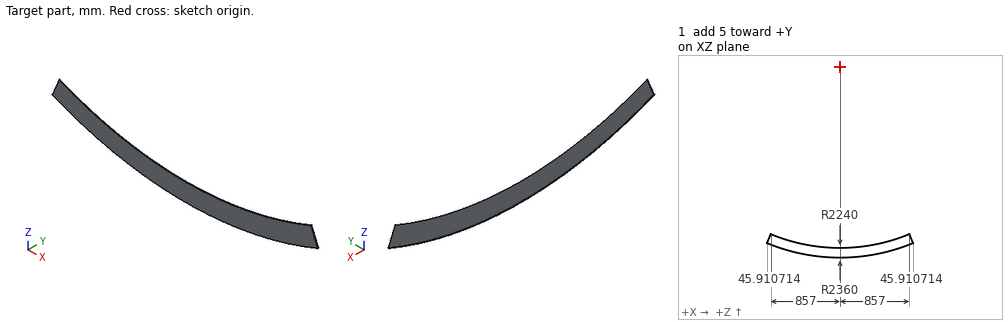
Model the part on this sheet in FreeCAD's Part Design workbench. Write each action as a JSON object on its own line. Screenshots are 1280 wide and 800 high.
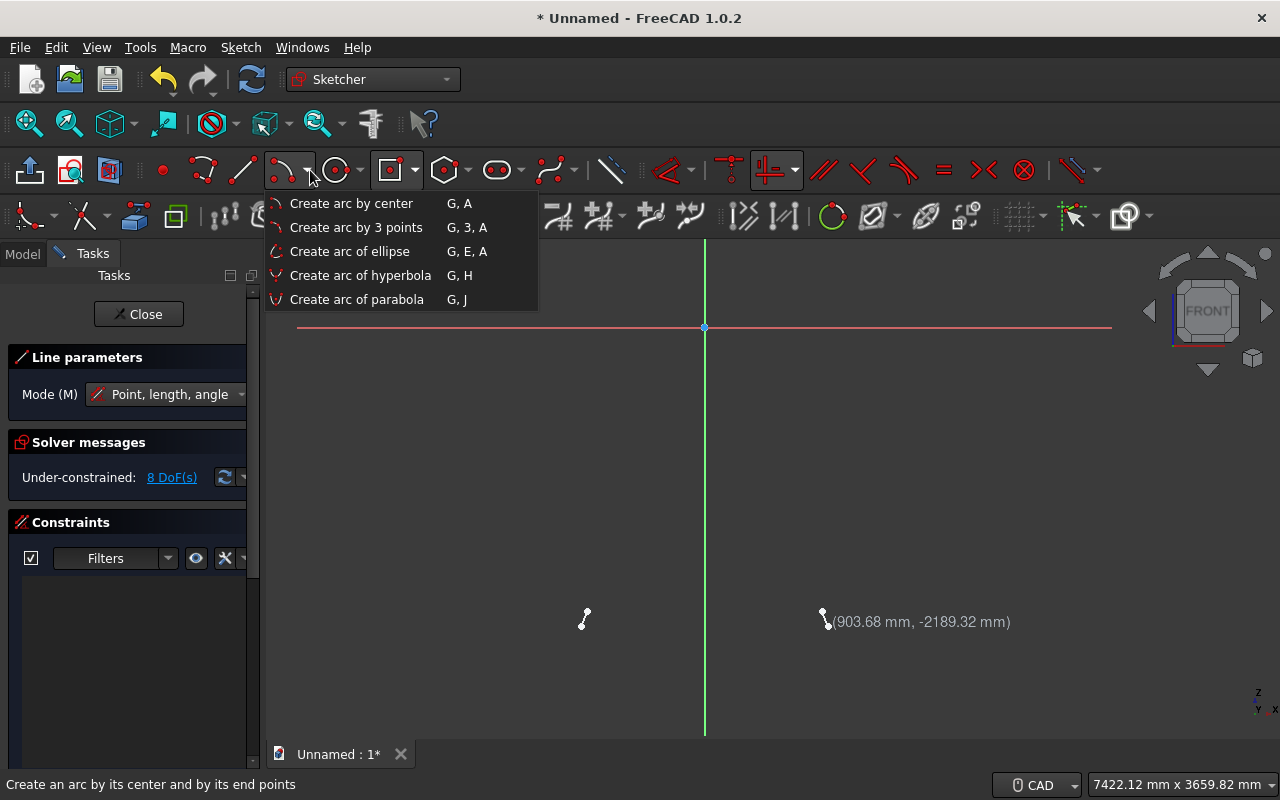
{"action": "left_click", "coordinate": [402, 227]}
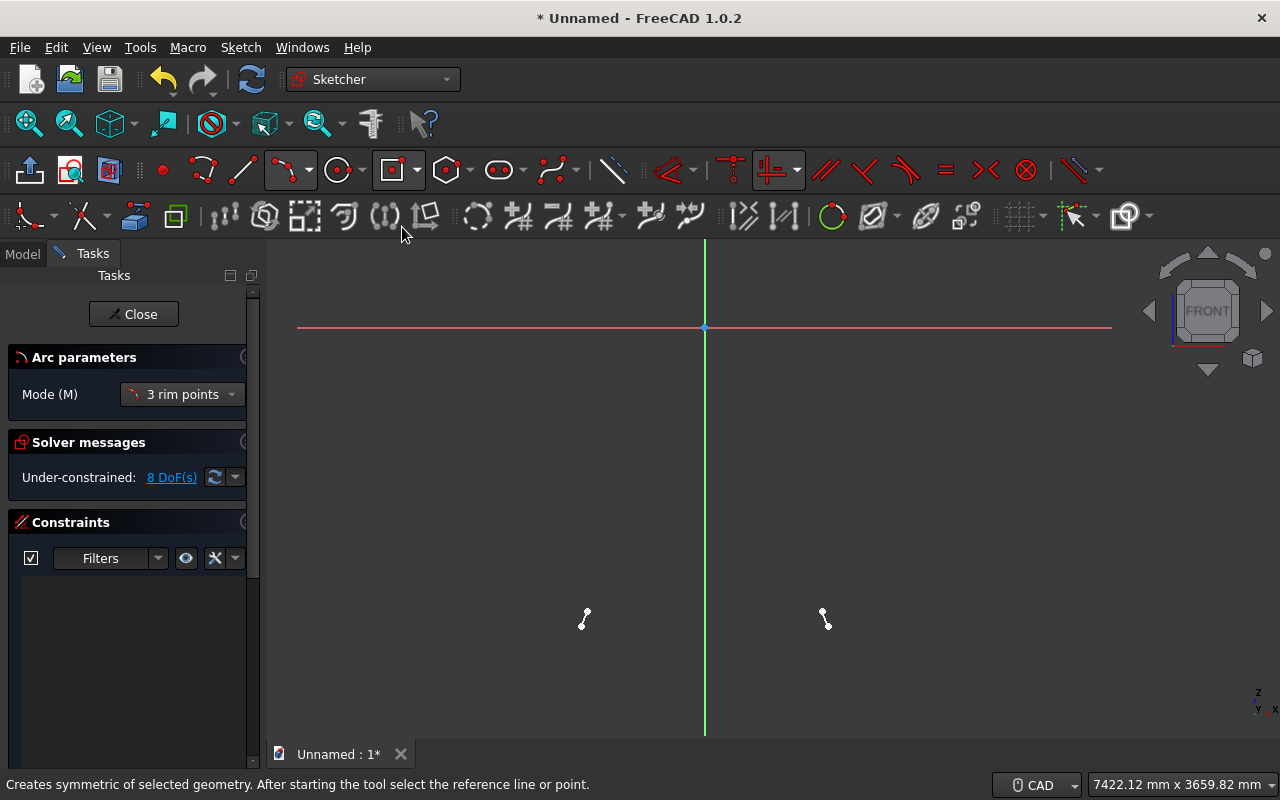
{"action": "scroll", "coordinate": [587, 611], "scroll_direction": "up", "scroll_amount": 4}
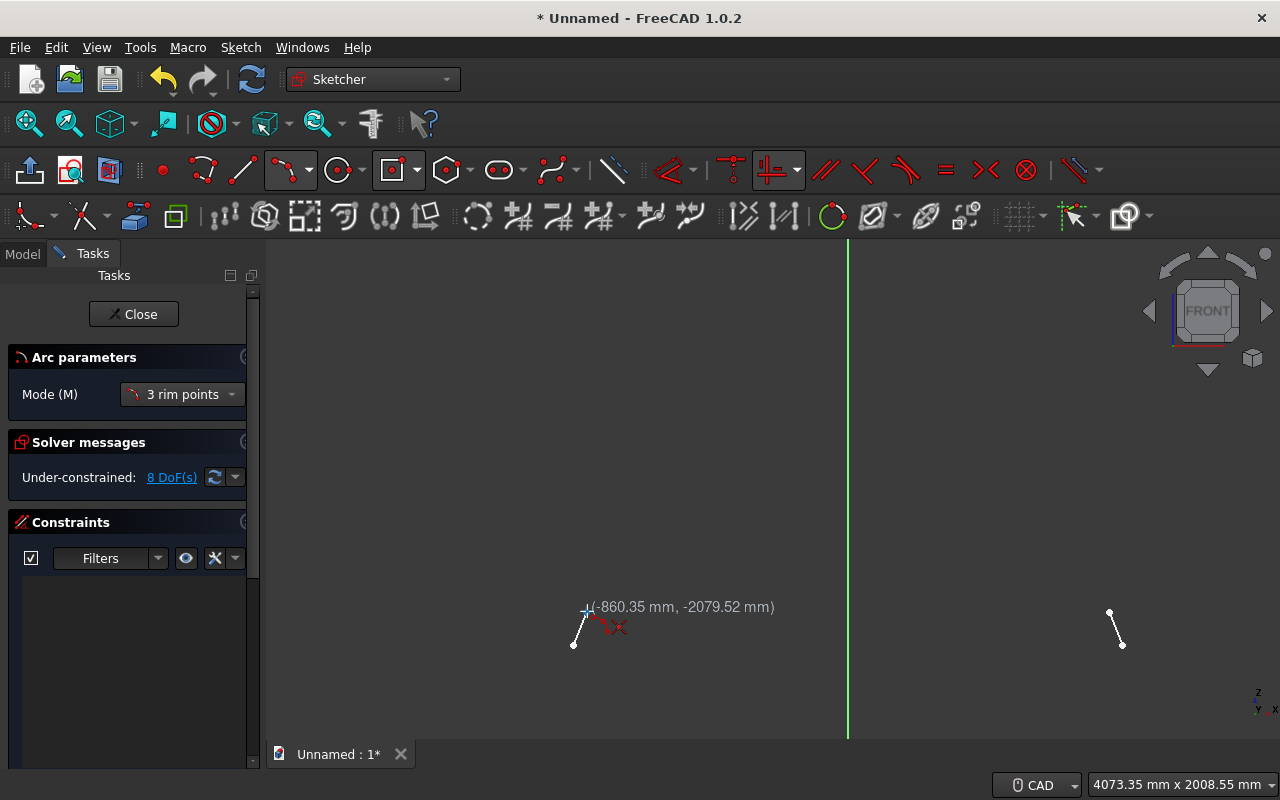
{"action": "left_click", "coordinate": [587, 612]}
{"action": "left_click", "coordinate": [1110, 612]}
{"action": "left_click", "coordinate": [795, 659]}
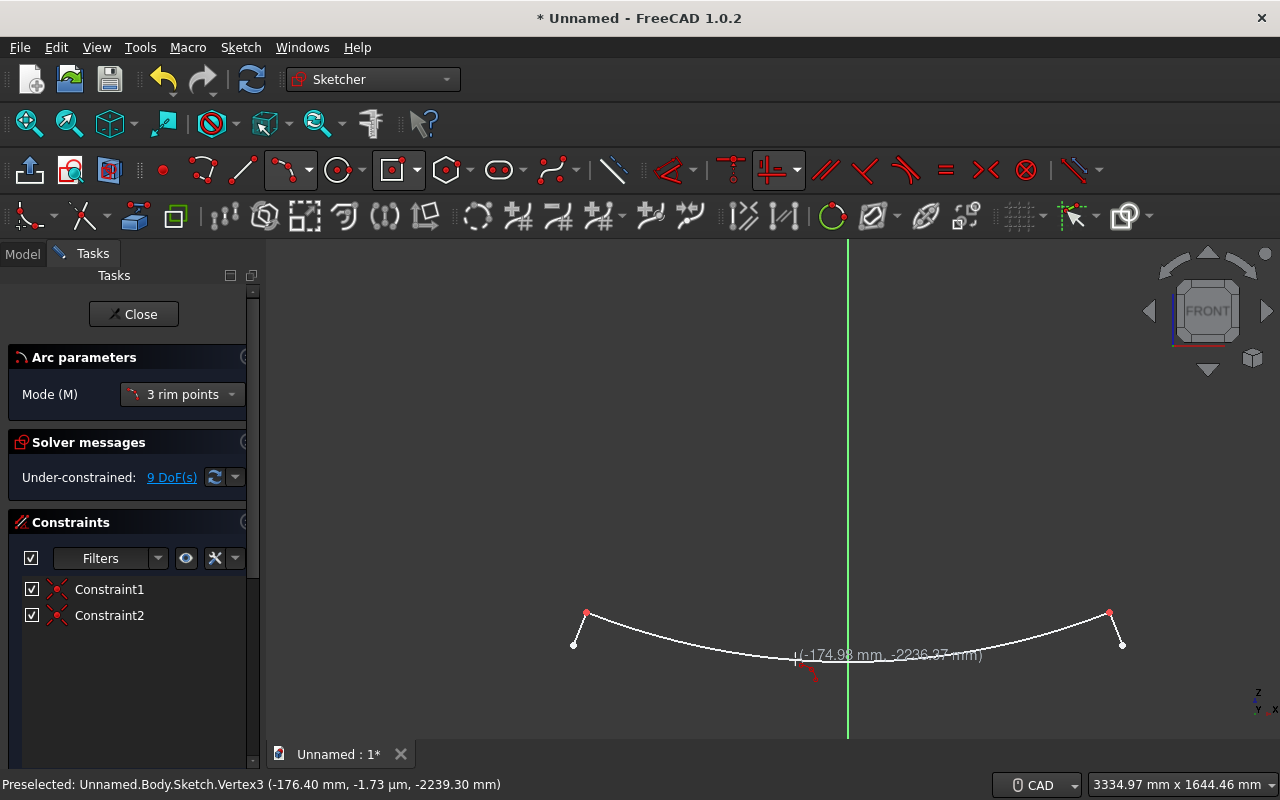
{"action": "scroll", "coordinate": [587, 612], "scroll_direction": "down", "scroll_amount": 4}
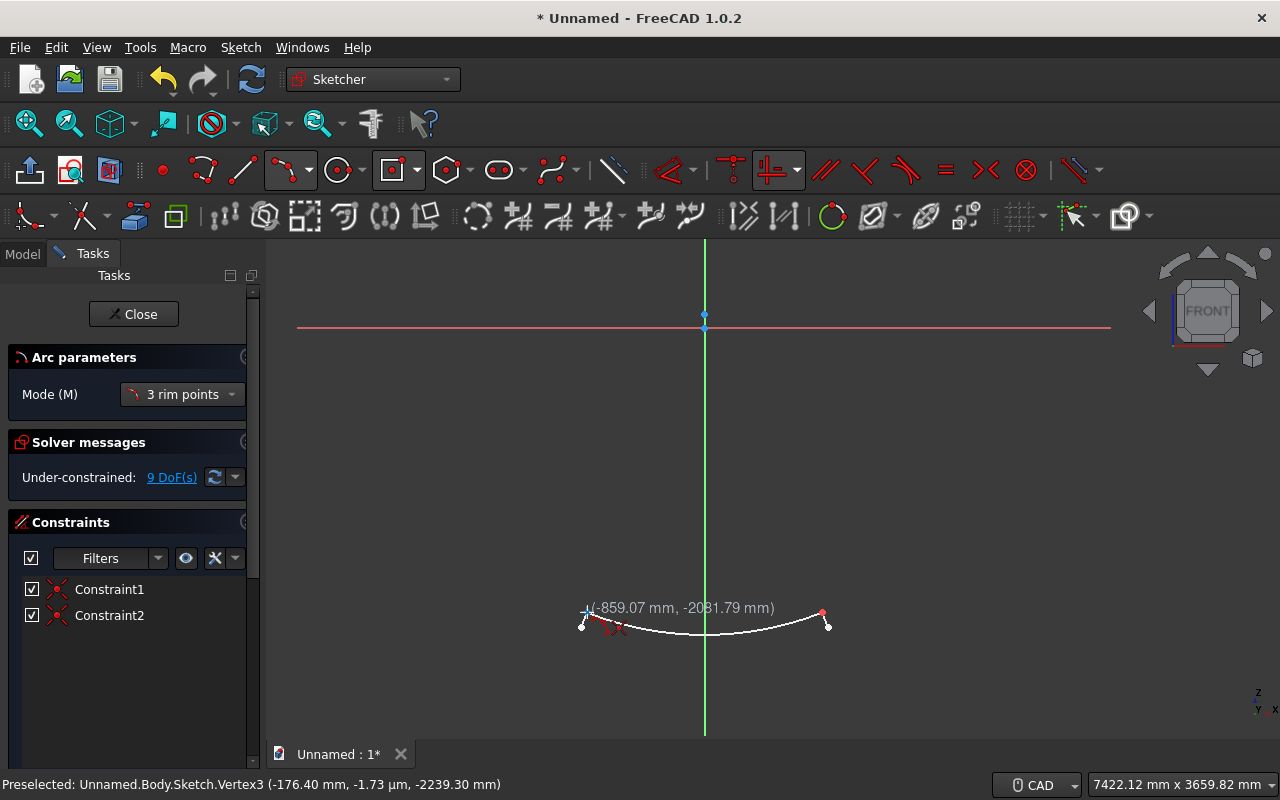
{"action": "scroll", "coordinate": [828, 626], "scroll_direction": "up", "scroll_amount": 4}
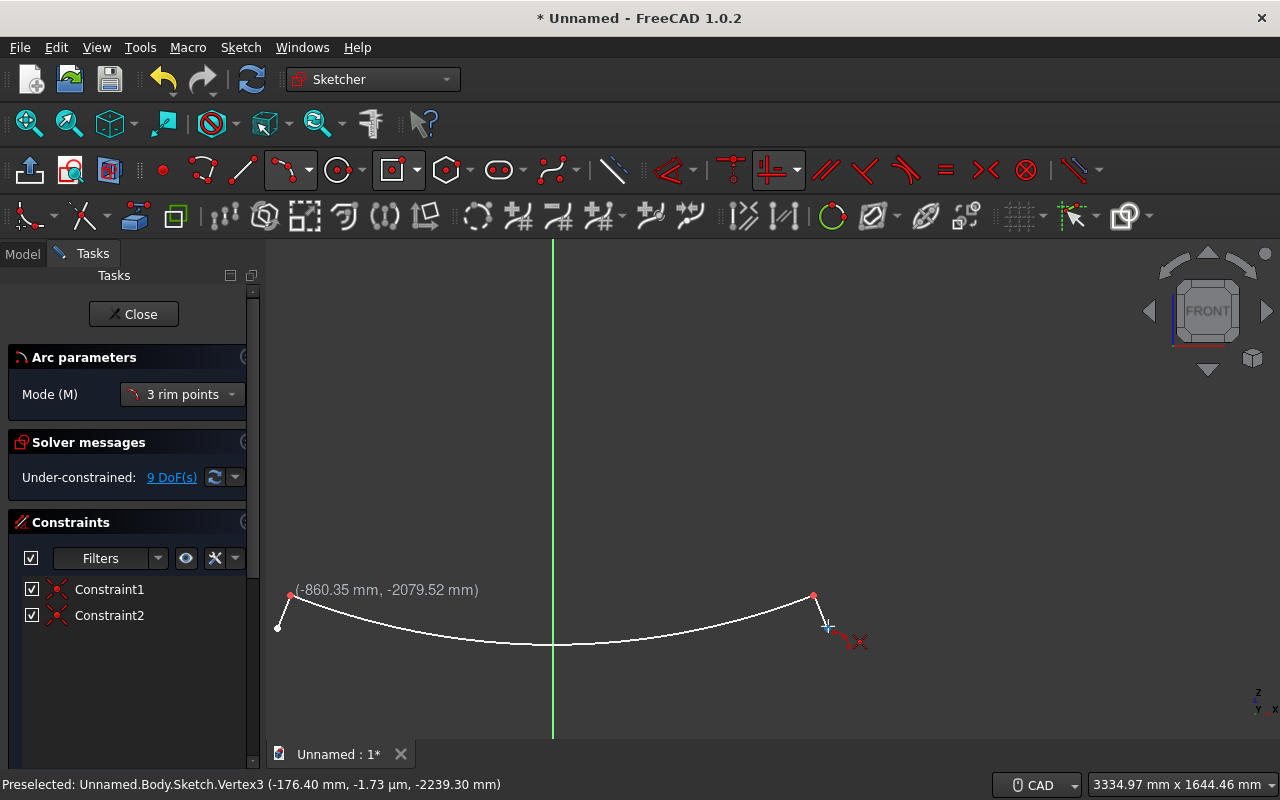
{"action": "left_click", "coordinate": [827, 629]}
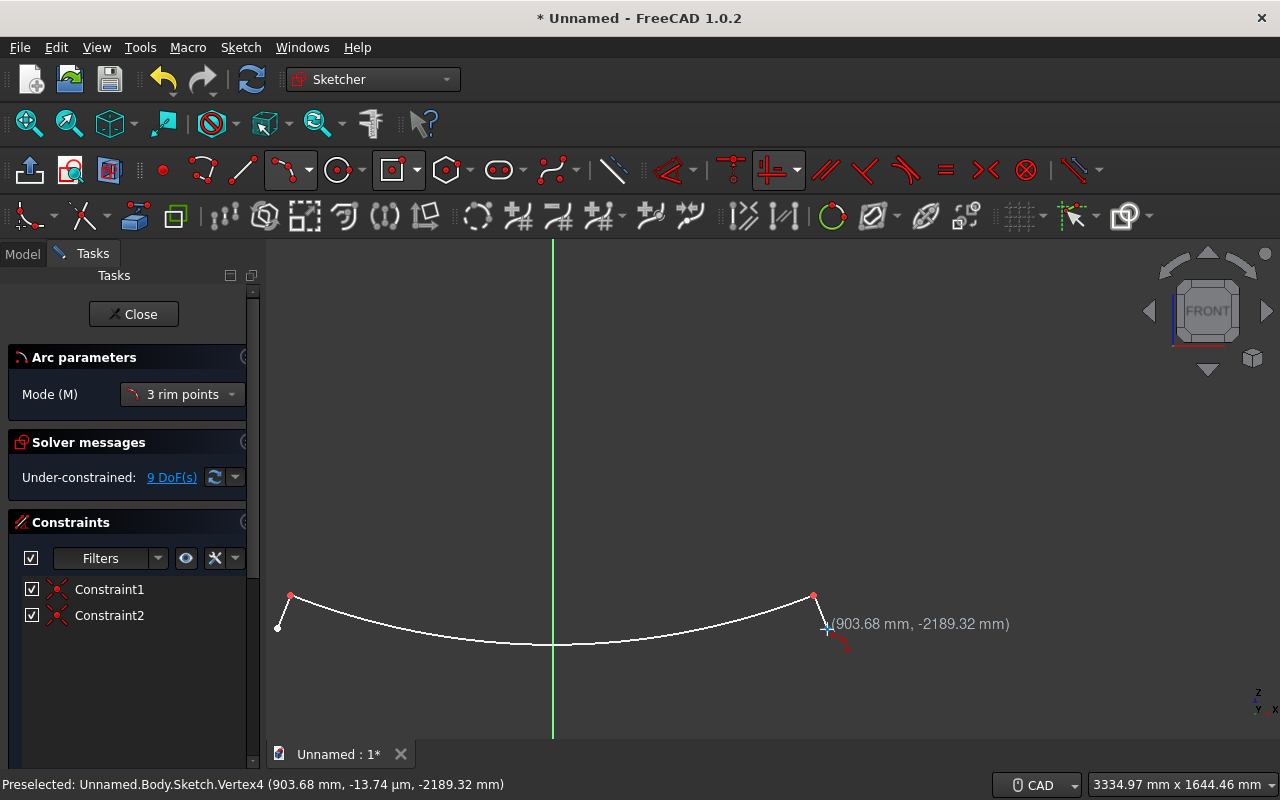
{"action": "scroll", "coordinate": [828, 626], "scroll_direction": "down", "scroll_amount": 4}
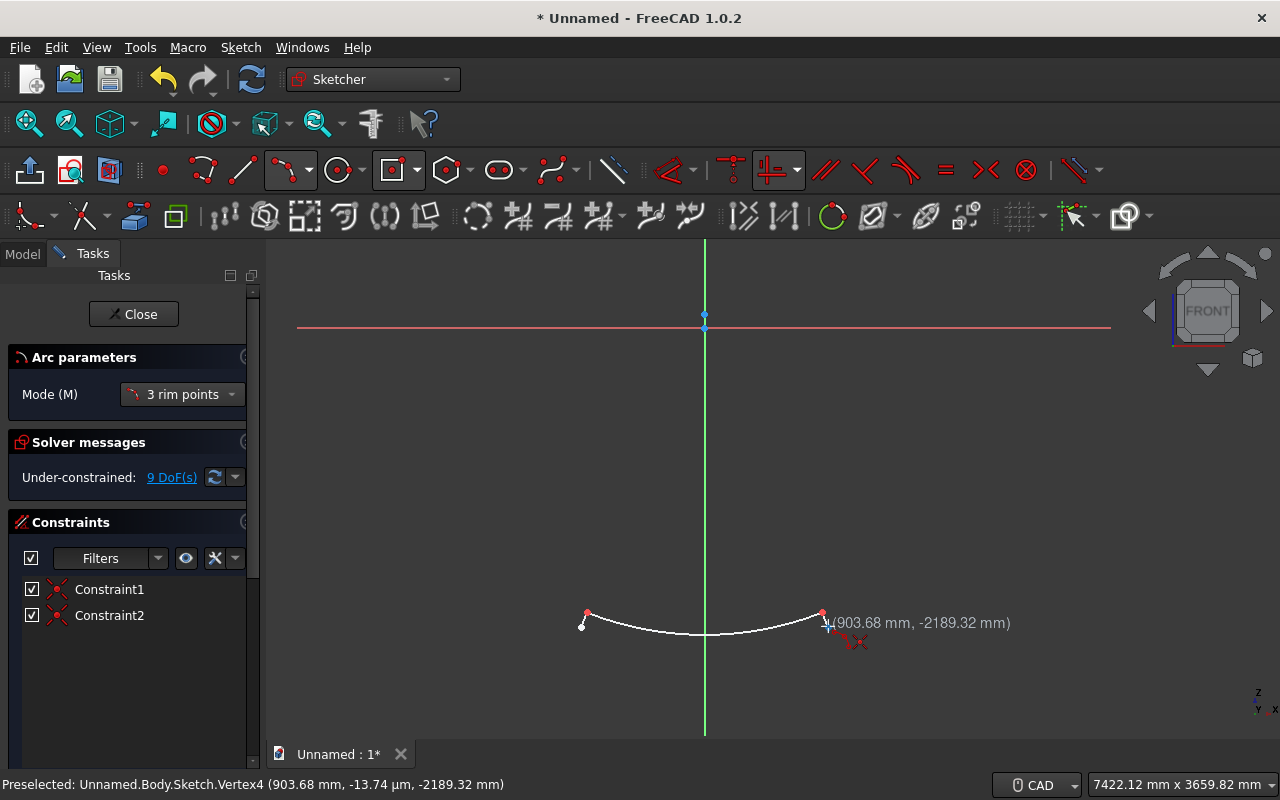
{"action": "scroll", "coordinate": [581, 626], "scroll_direction": "up", "scroll_amount": 4}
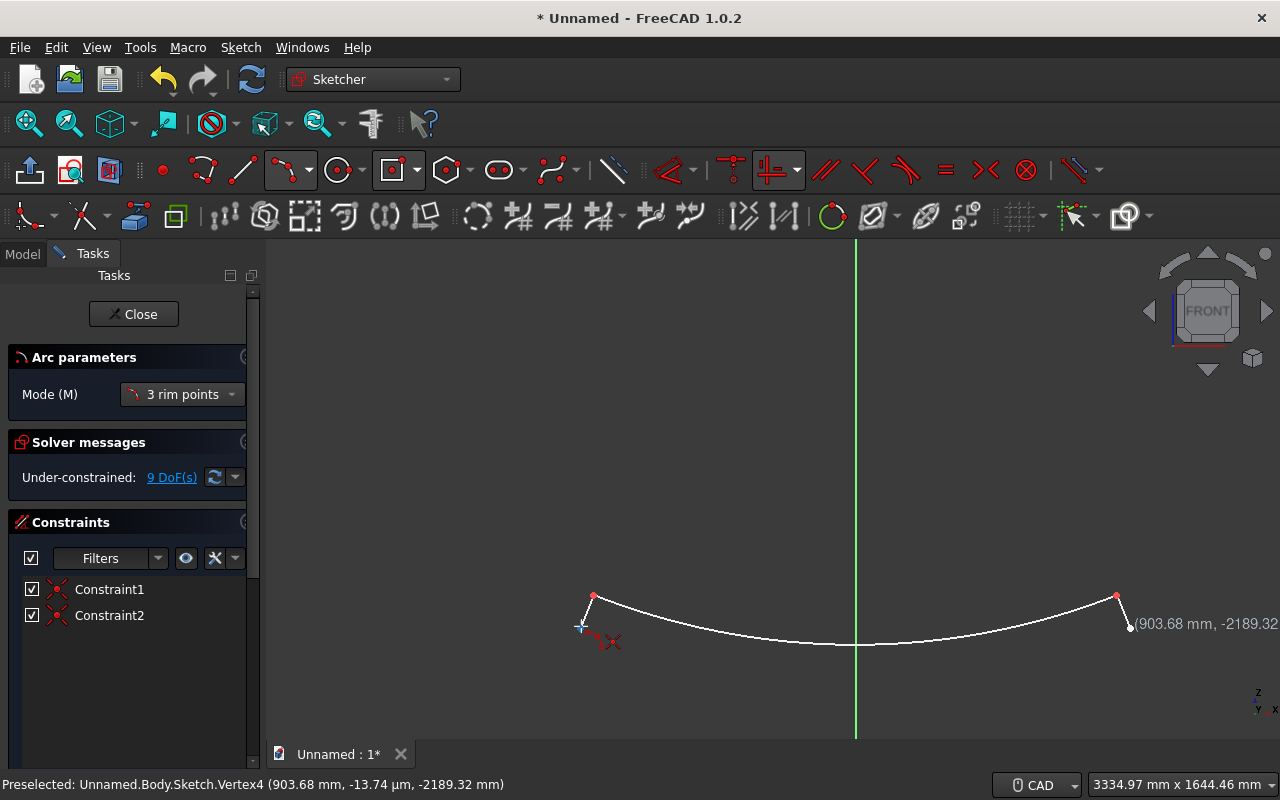
{"action": "left_click", "coordinate": [581, 629]}
{"action": "left_click", "coordinate": [799, 678]}
{"action": "key", "text": "Escape"}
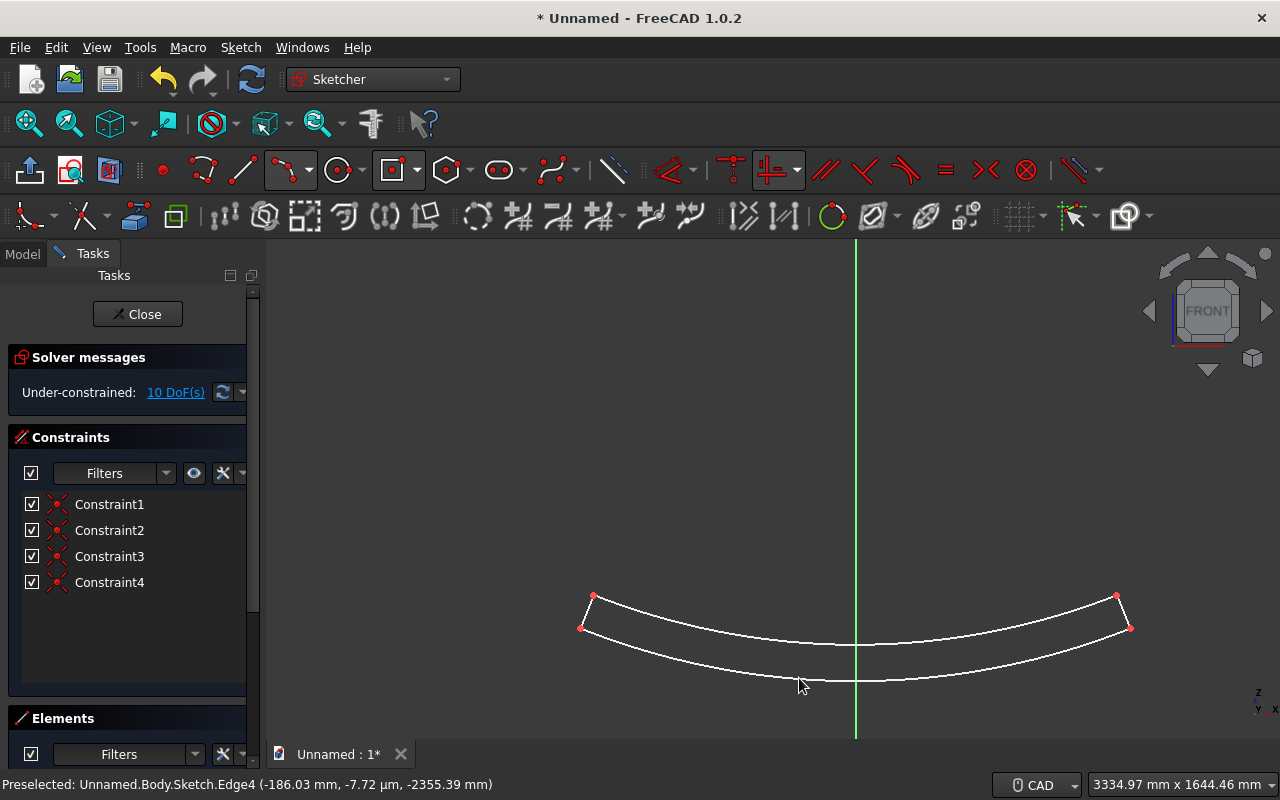
{"action": "left_click", "coordinate": [749, 637]}